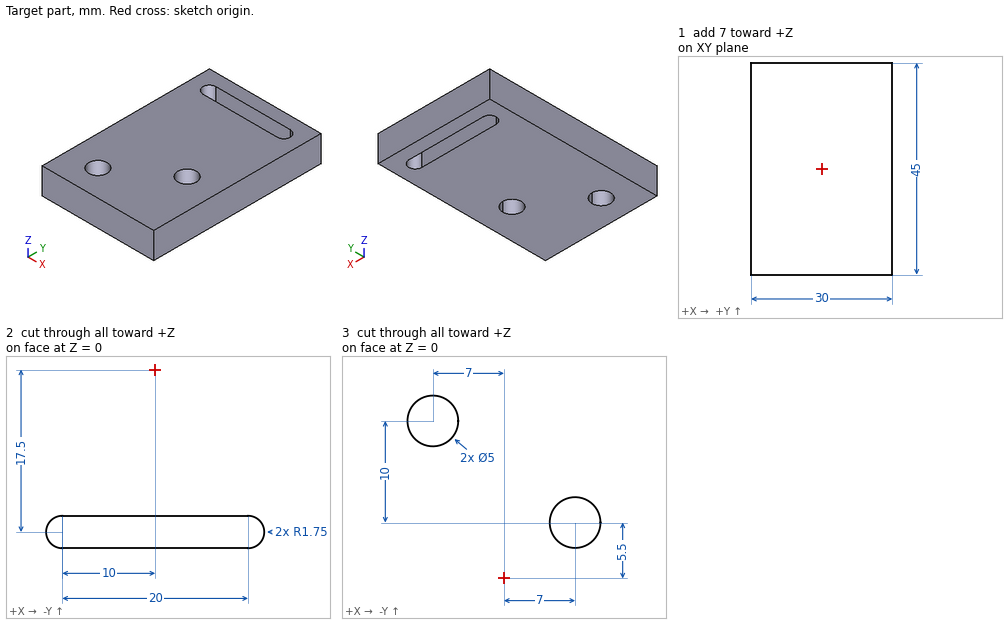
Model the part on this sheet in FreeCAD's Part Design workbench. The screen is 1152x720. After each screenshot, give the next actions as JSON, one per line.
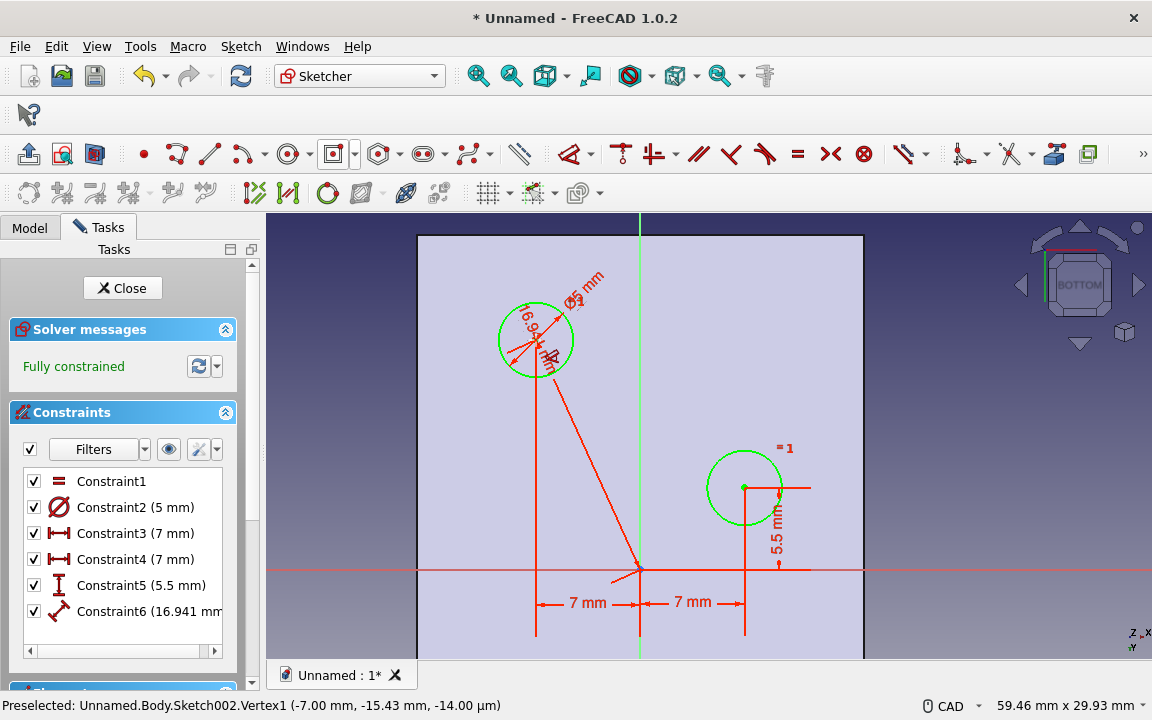
{"action": "left_click", "coordinate": [745, 488]}
{"action": "left_click", "coordinate": [779, 414]}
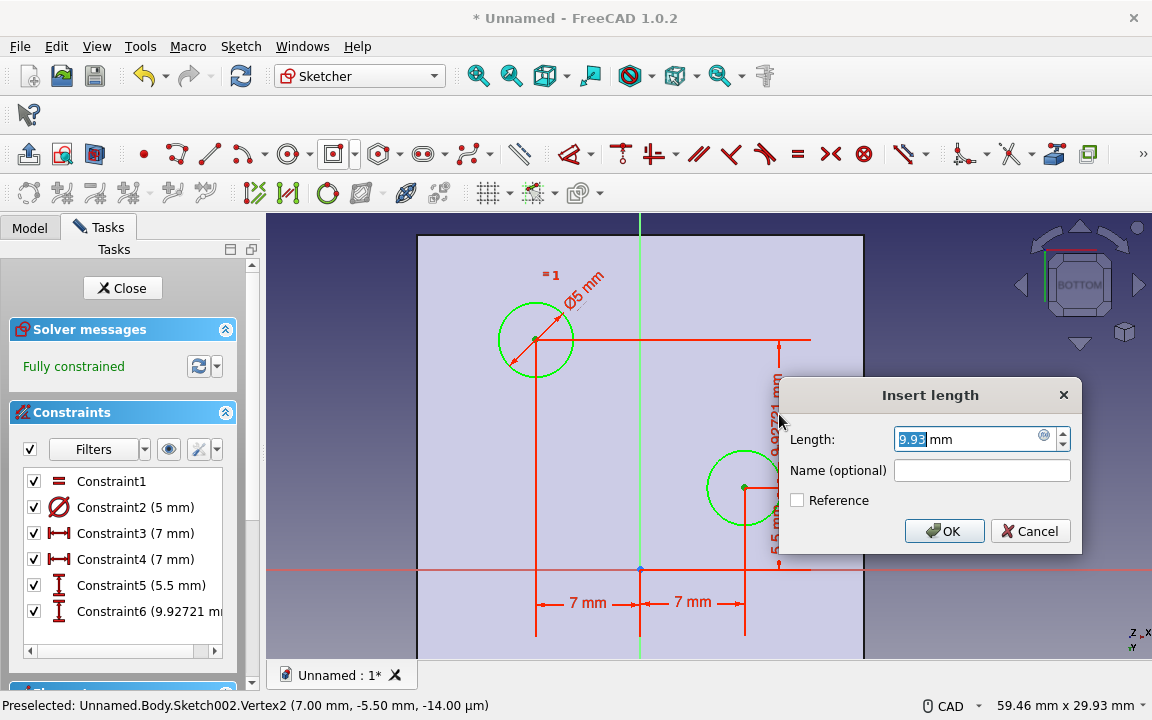
{"action": "type", "text": "10"}
{"action": "key", "text": "Return"}
{"action": "key", "text": "Escape"}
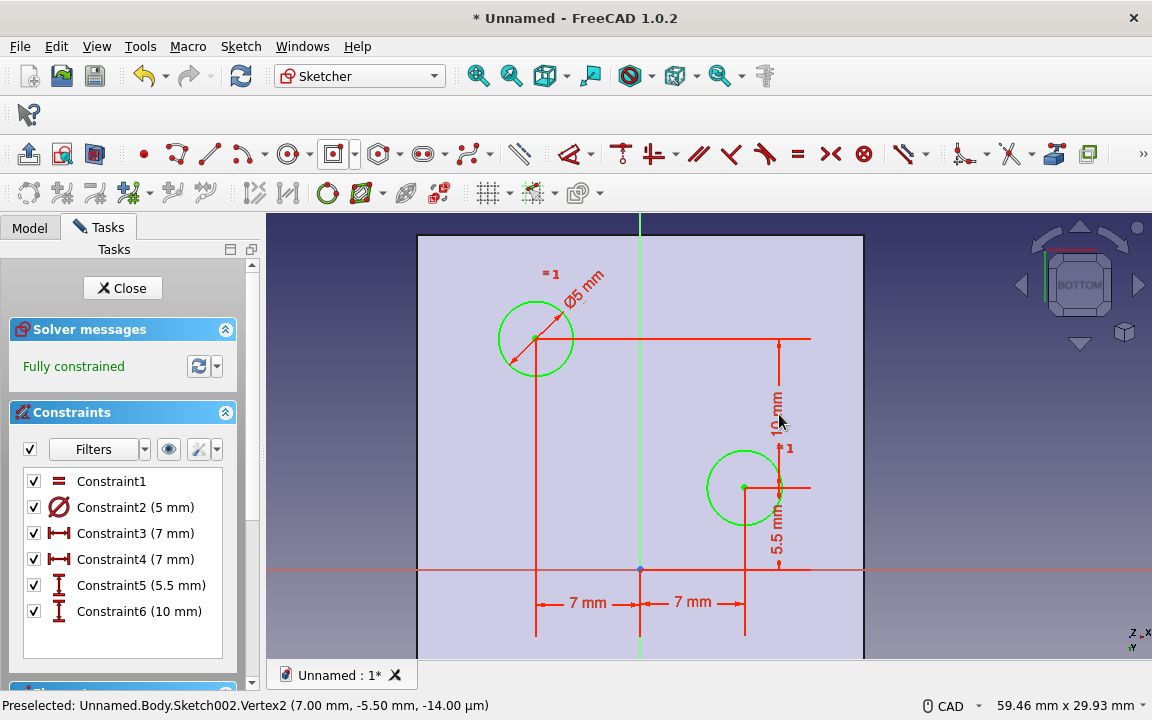
{"action": "left_click", "coordinate": [123, 288]}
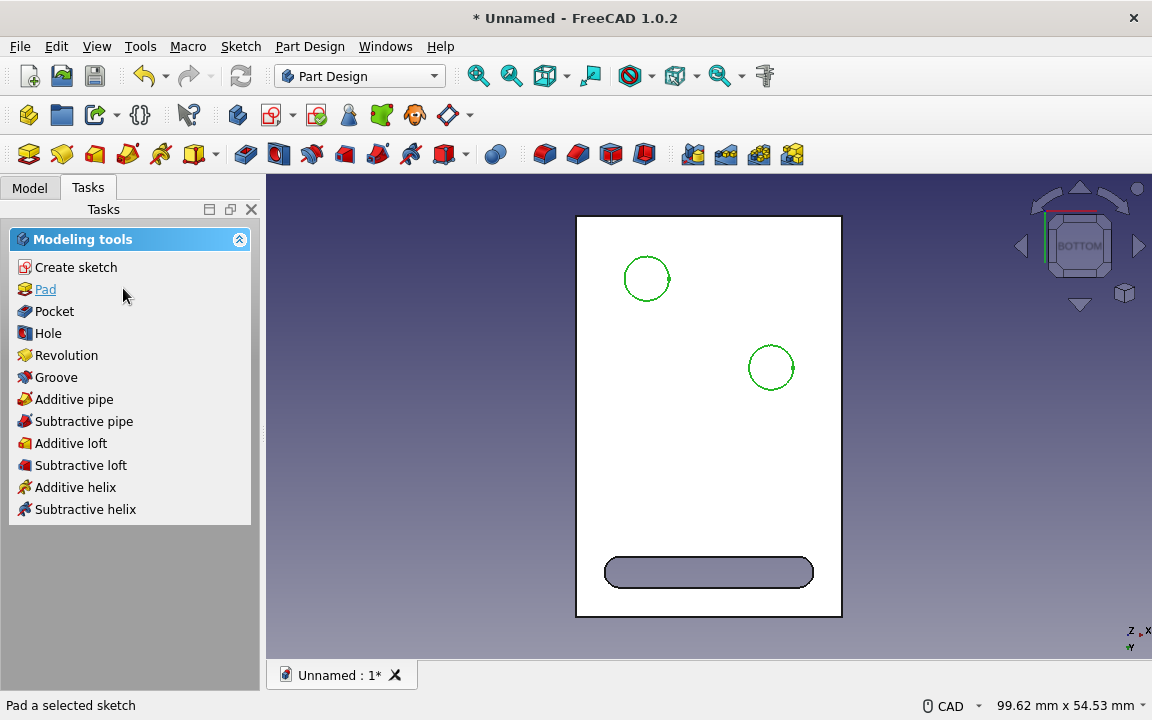
{"action": "left_click", "coordinate": [246, 154]}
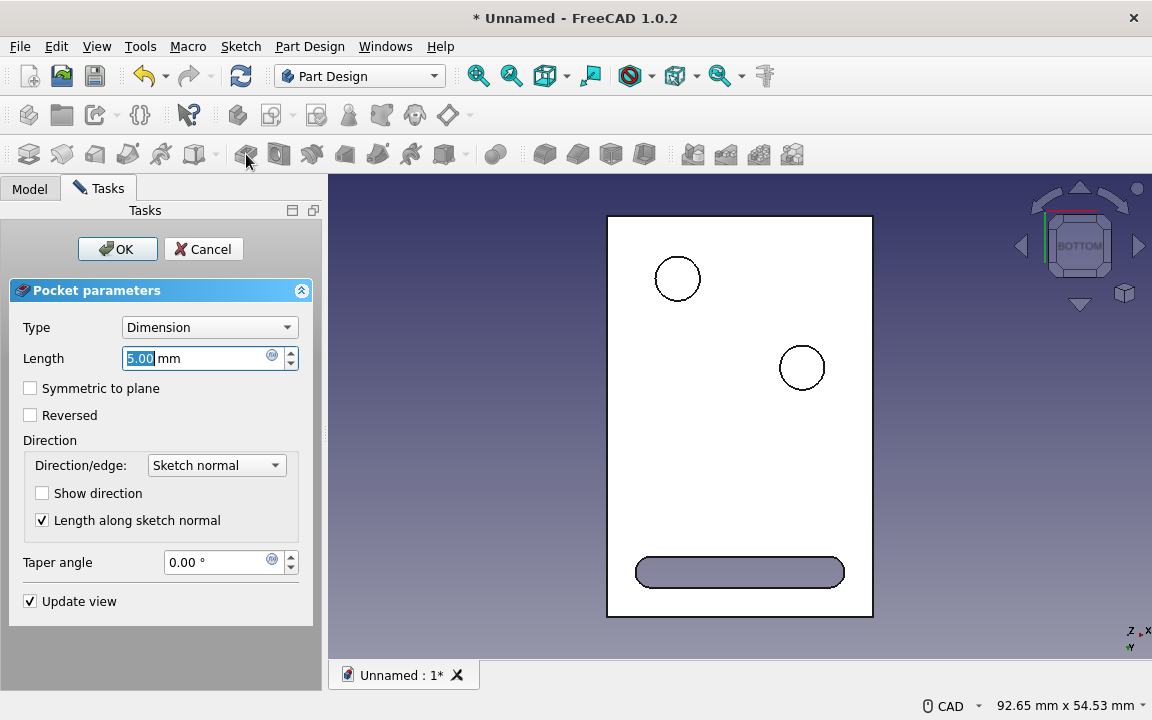
{"action": "left_click", "coordinate": [210, 328]}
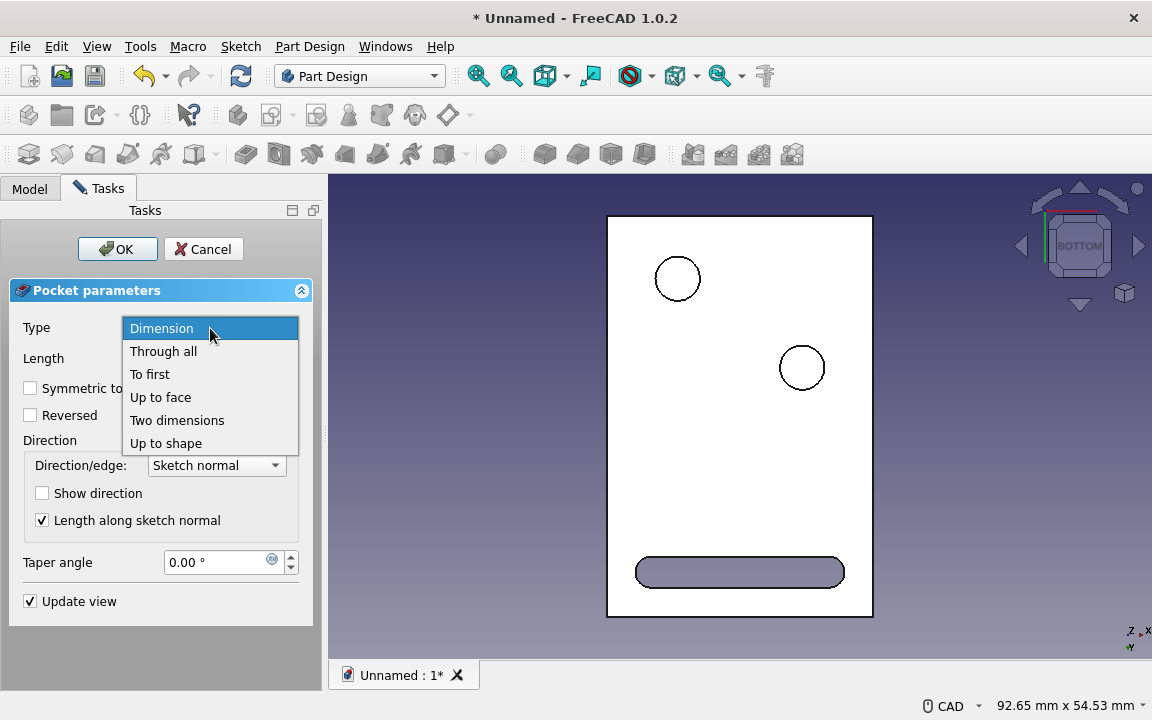
{"action": "left_click", "coordinate": [208, 352]}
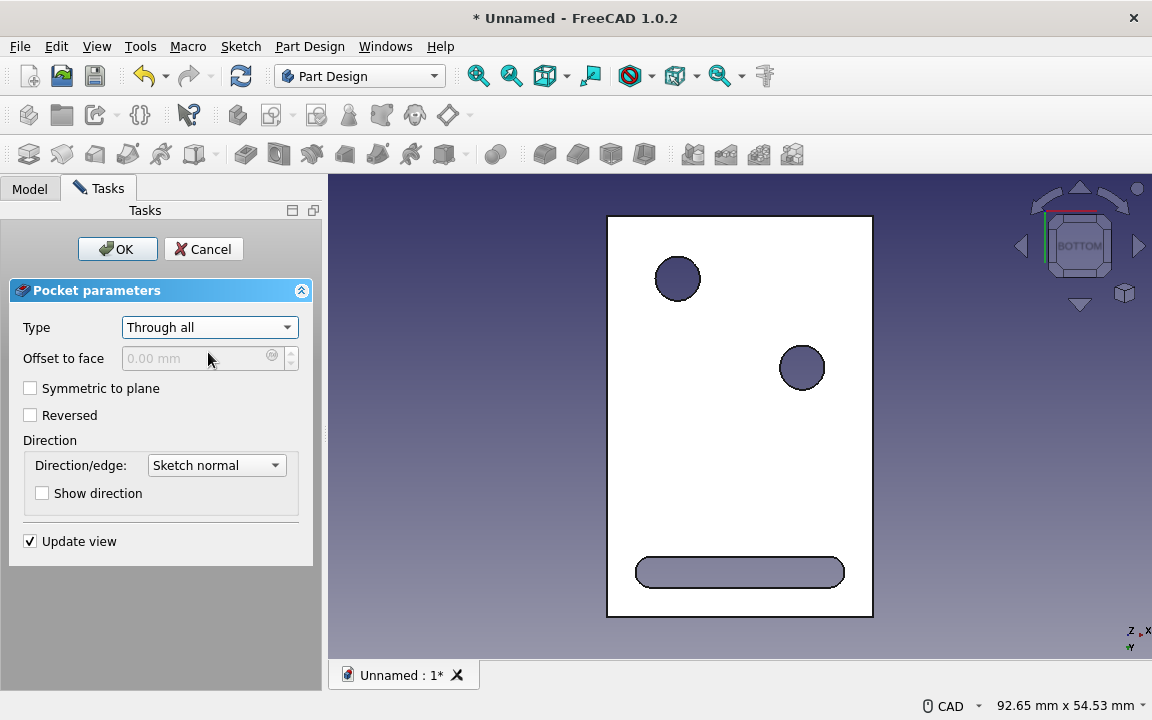
{"action": "left_click", "coordinate": [118, 249]}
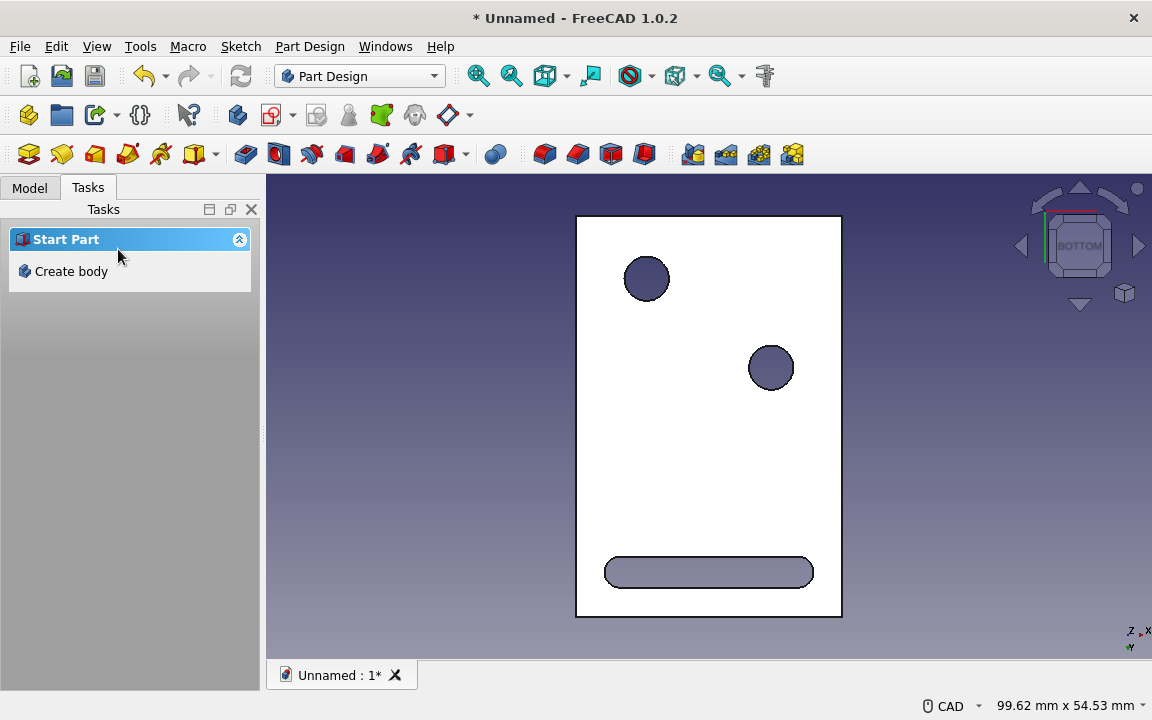
{"action": "key", "text": "0"}